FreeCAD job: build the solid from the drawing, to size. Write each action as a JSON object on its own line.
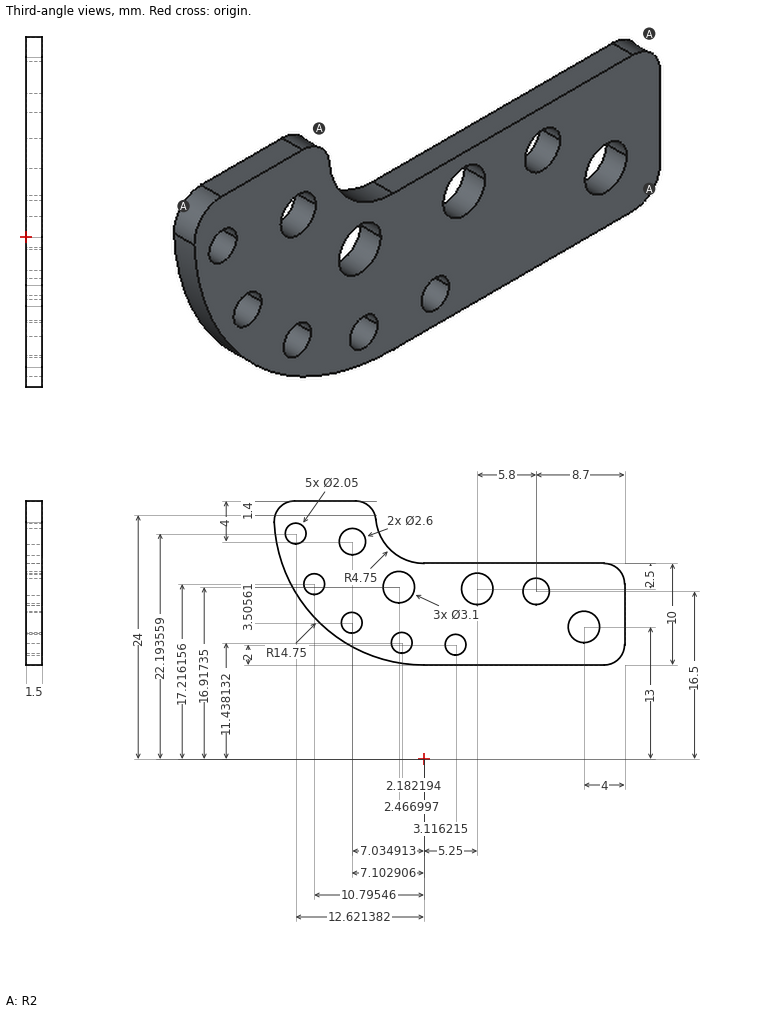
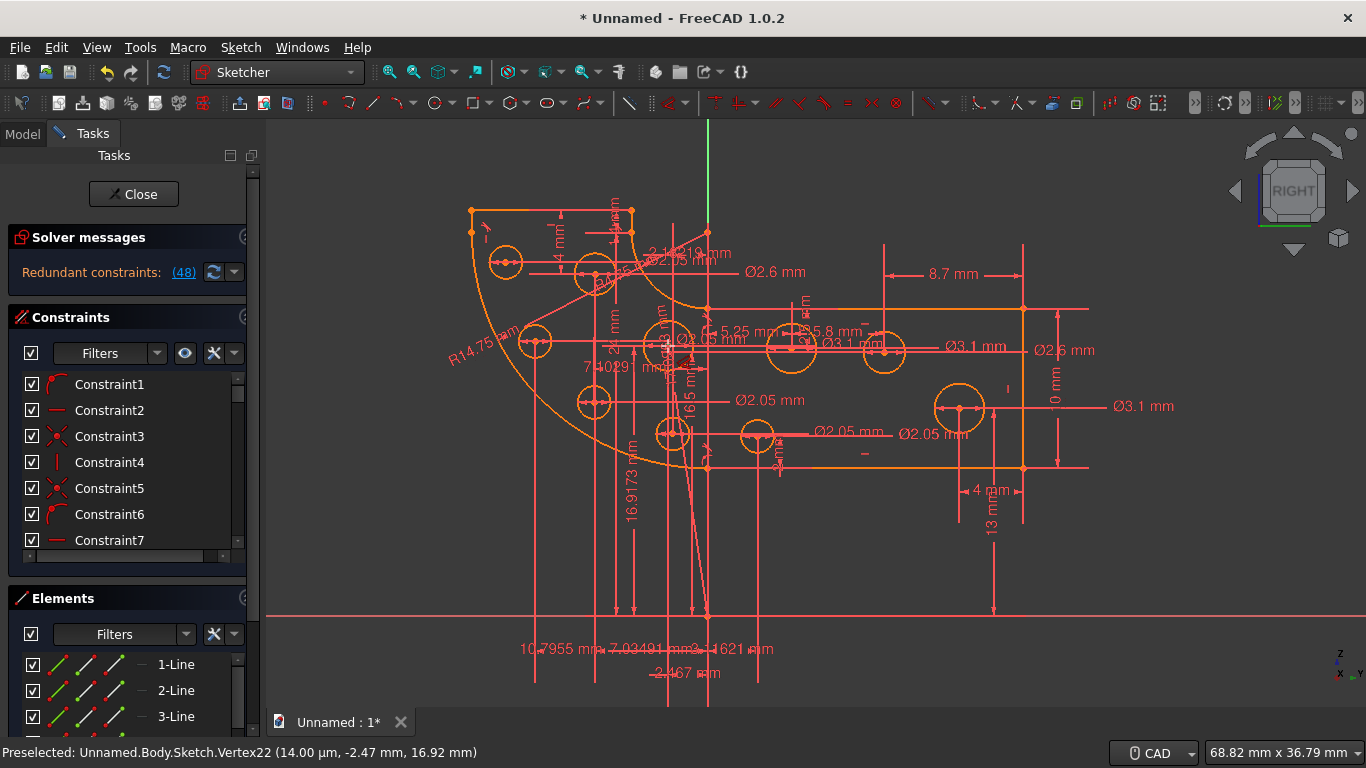
{"action": "left_click", "coordinate": [594, 402]}
{"action": "left_click", "coordinate": [560, 394]}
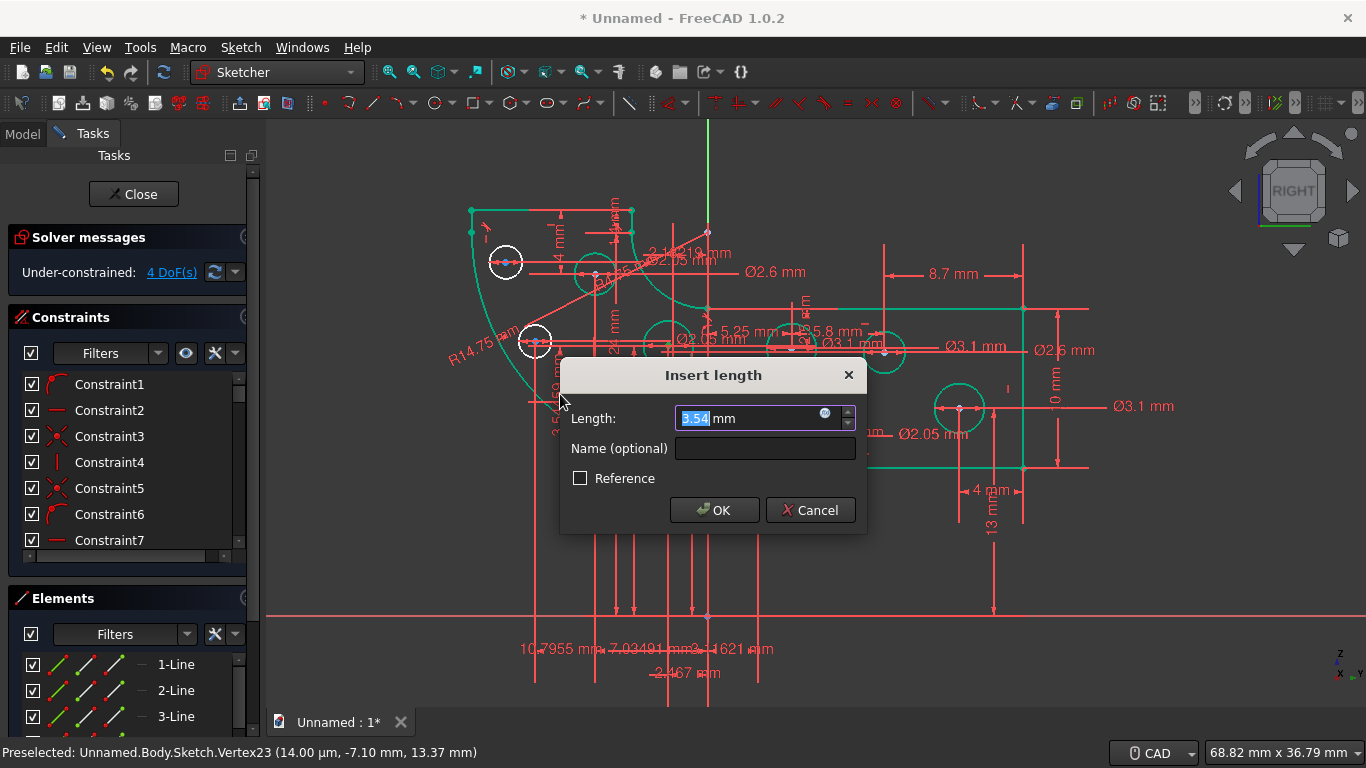
{"action": "type", "text": "3.50561"}
{"action": "key", "text": "Return"}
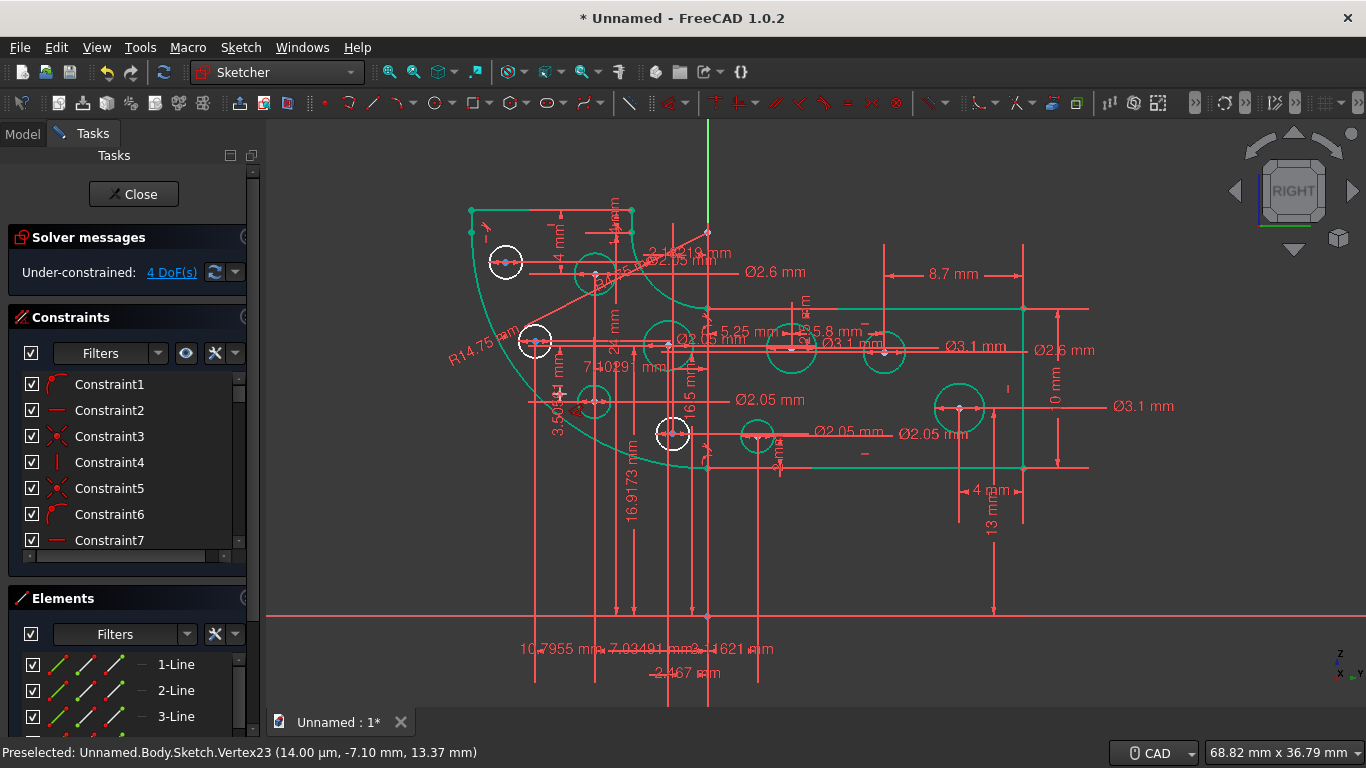
{"action": "left_click", "coordinate": [506, 262]}
{"action": "left_click", "coordinate": [607, 674]}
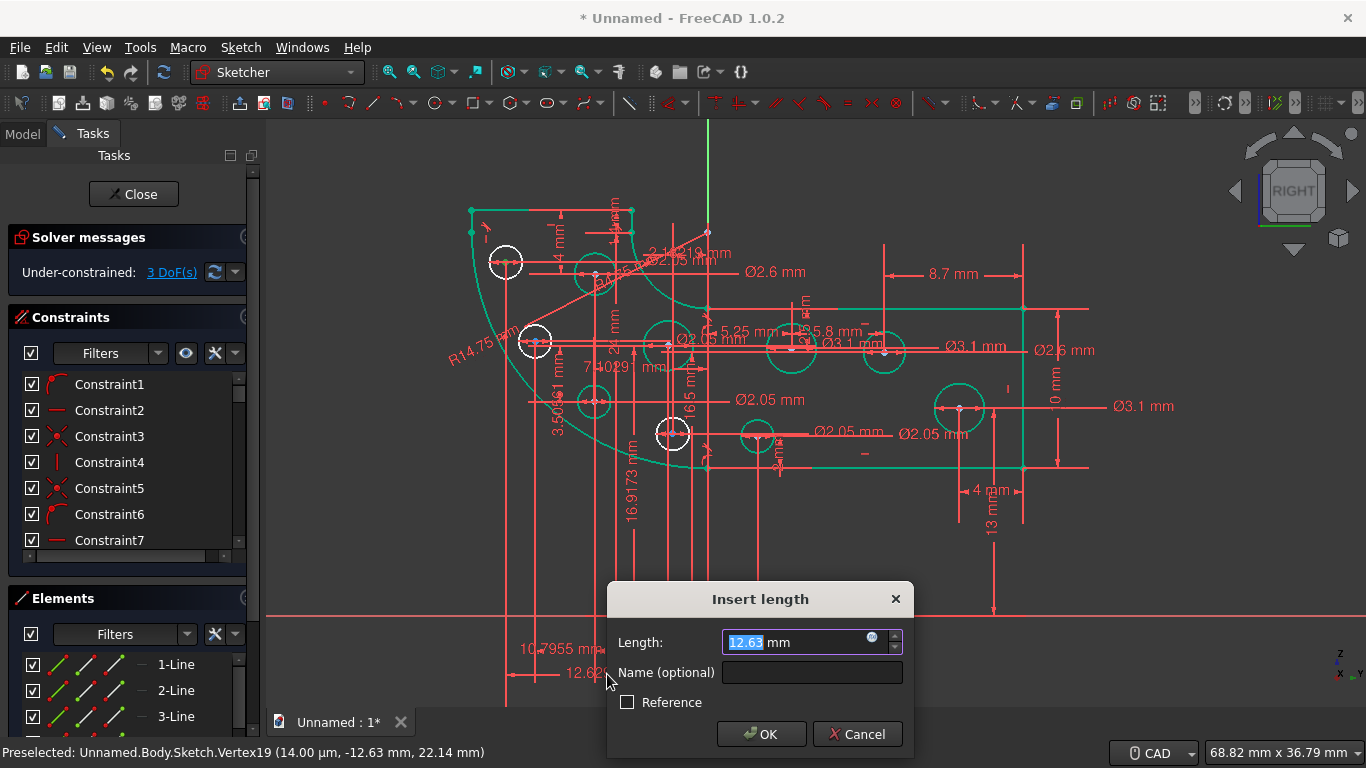
{"action": "type", "text": "12.621382"}
{"action": "key", "text": "Return"}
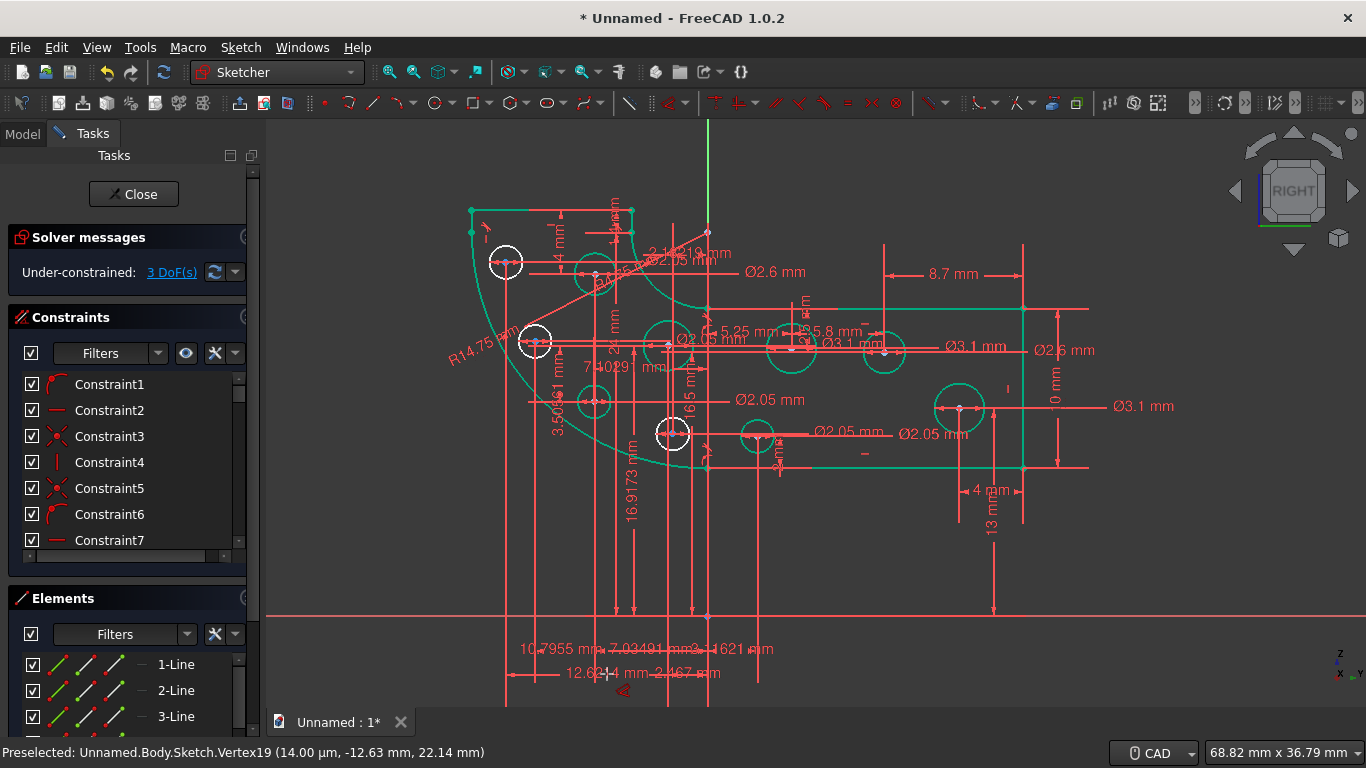
{"action": "left_click", "coordinate": [506, 262]}
{"action": "left_click", "coordinate": [472, 439]}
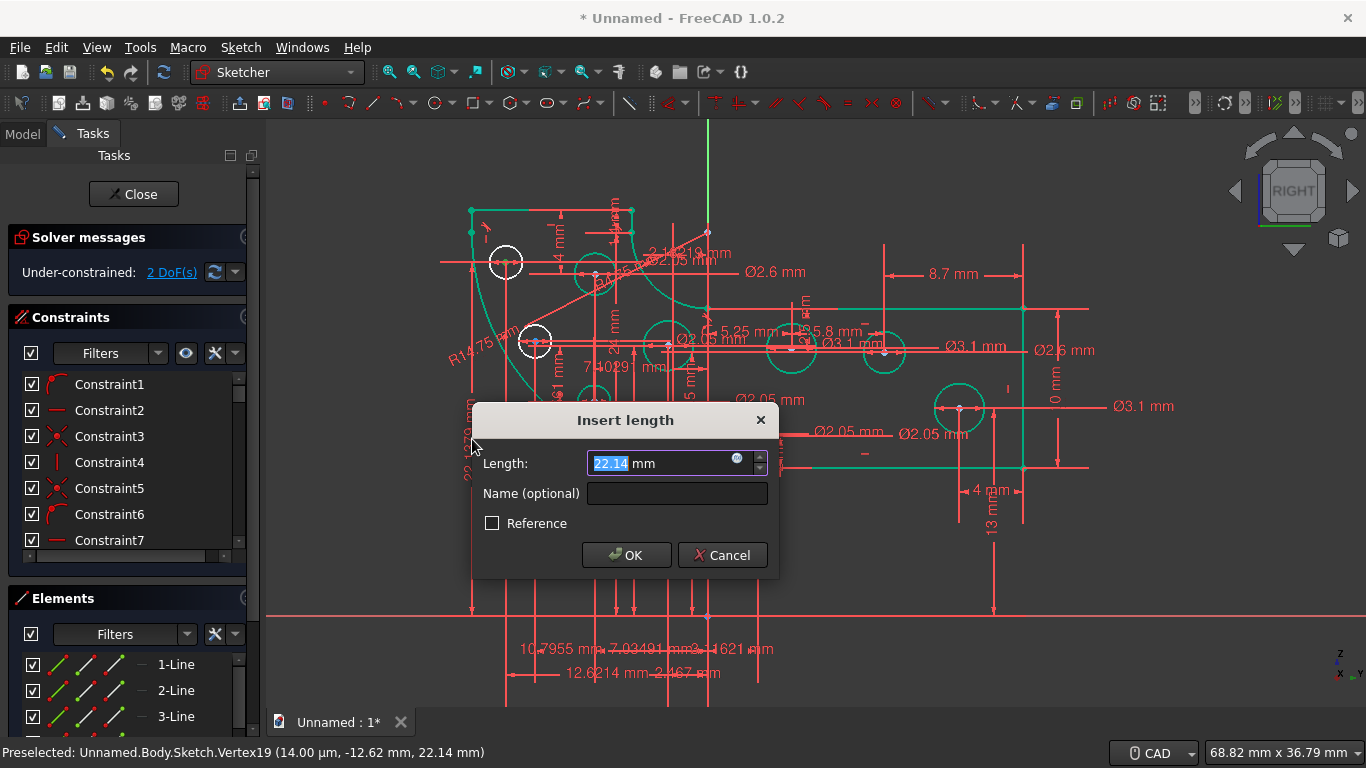
{"action": "type", "text": "22.193559"}
{"action": "key", "text": "Return"}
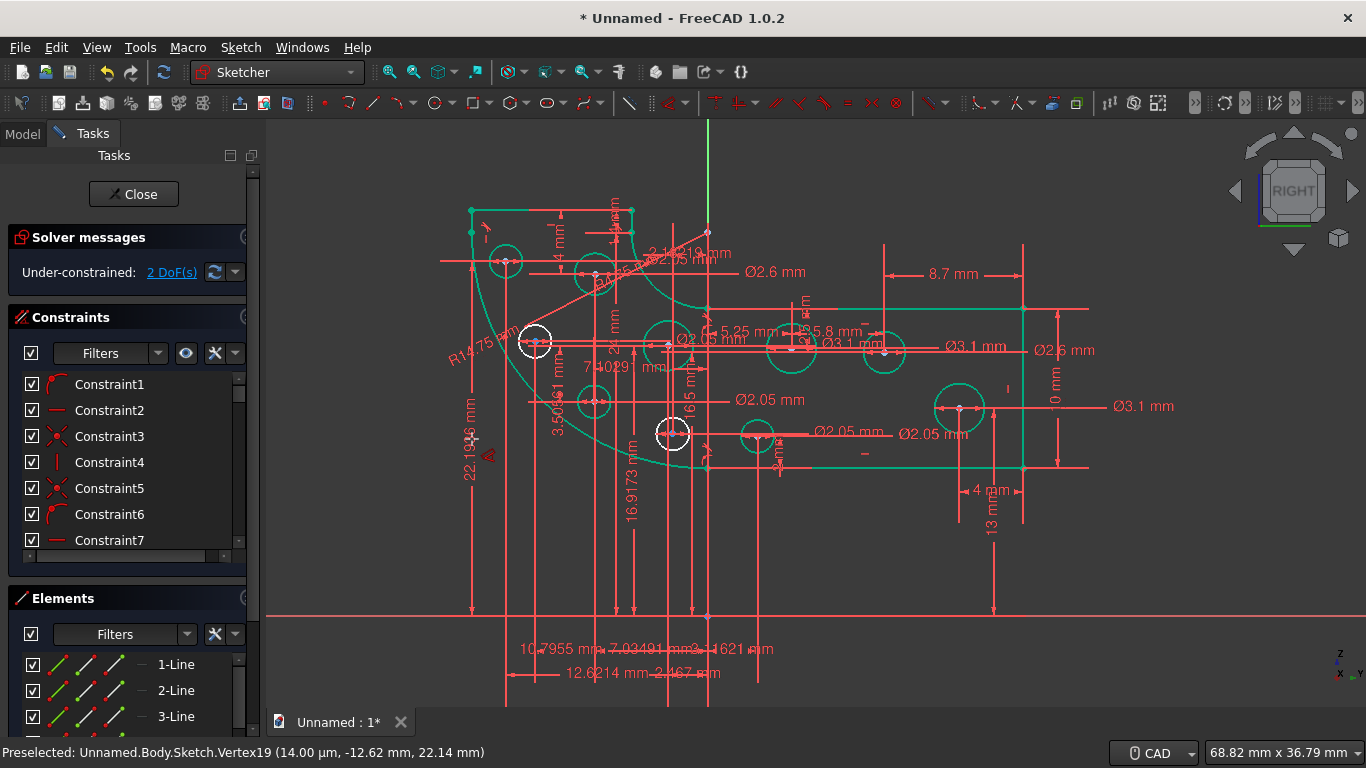
{"action": "left_click", "coordinate": [535, 341]}
{"action": "left_click", "coordinate": [501, 479]}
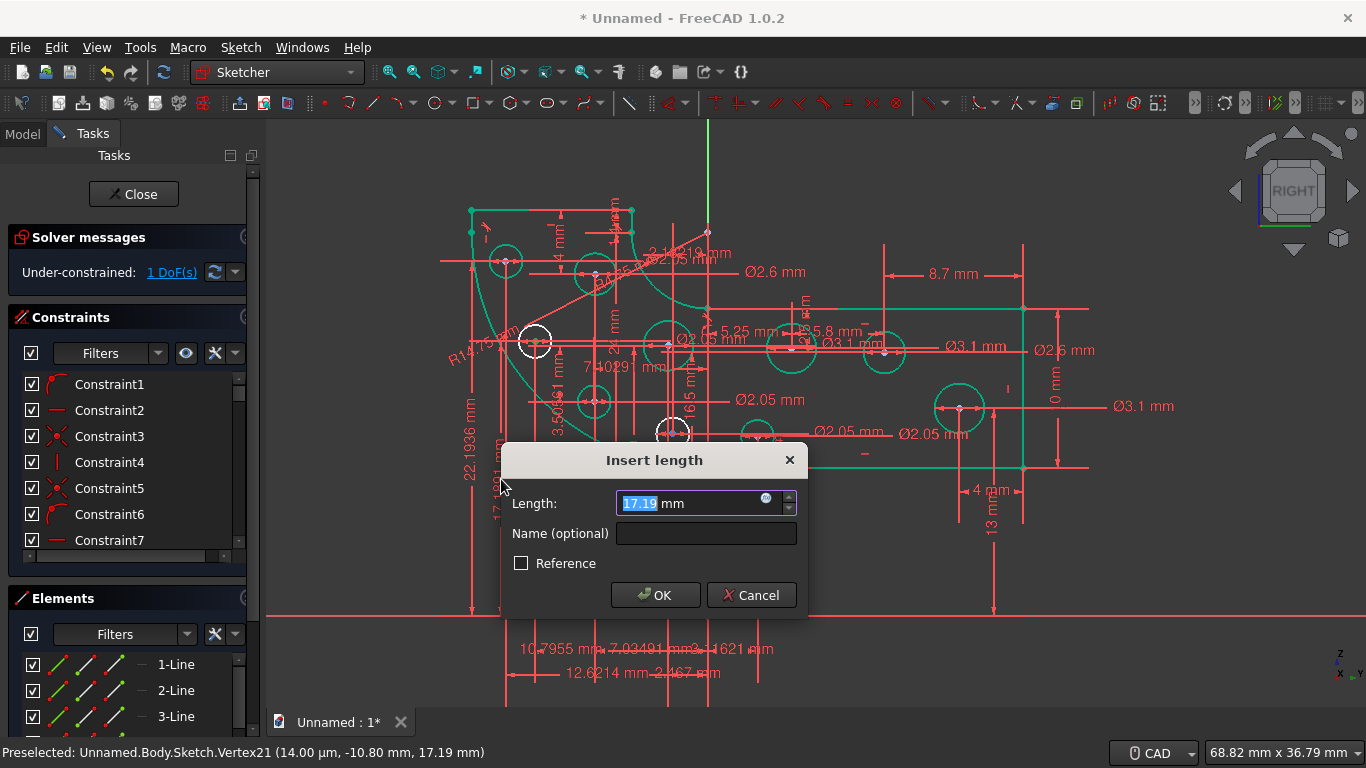
{"action": "type", "text": "17.216156"}
{"action": "key", "text": "Return"}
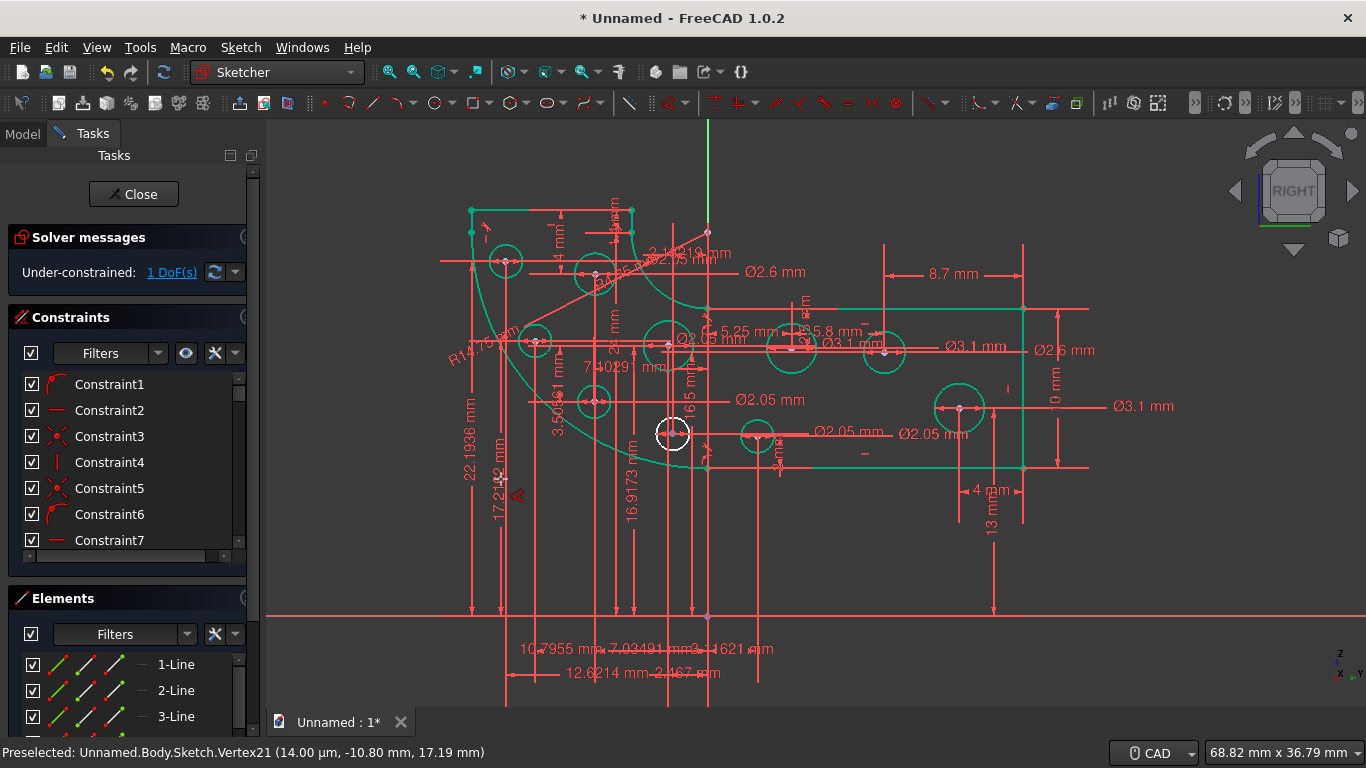
{"action": "left_click", "coordinate": [673, 434]}
{"action": "left_click", "coordinate": [639, 525]}